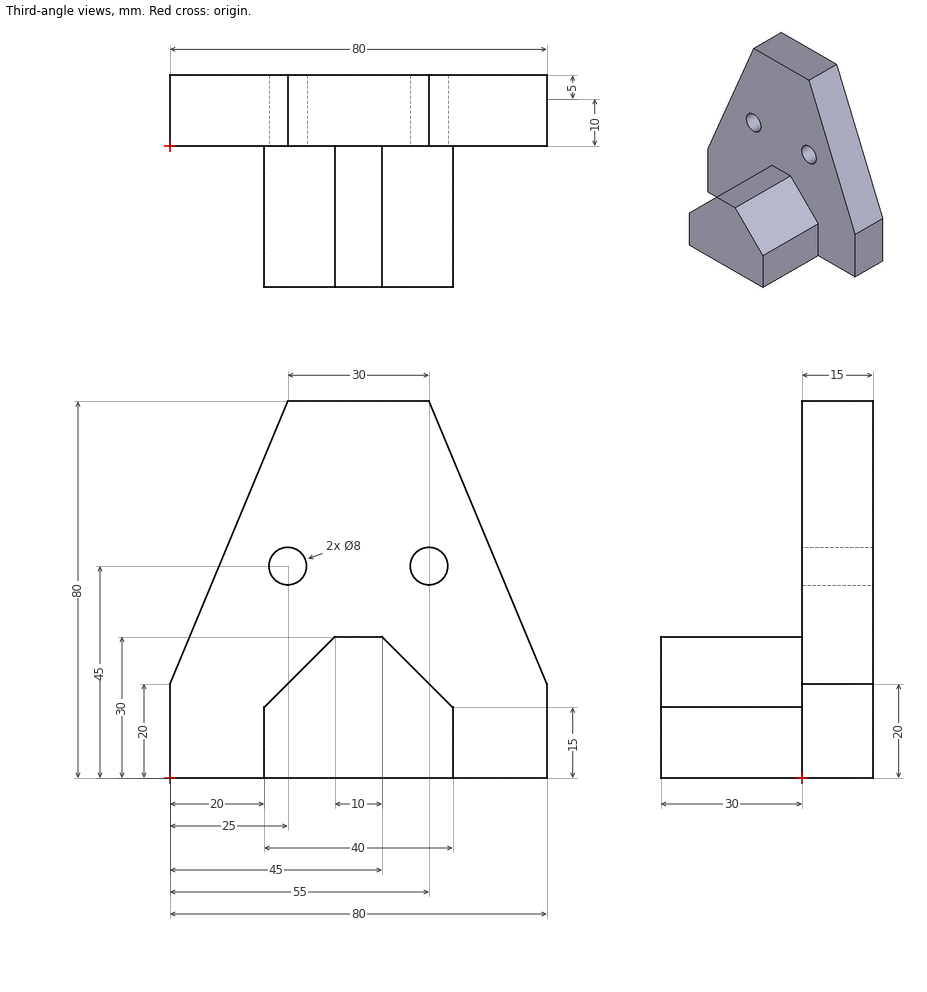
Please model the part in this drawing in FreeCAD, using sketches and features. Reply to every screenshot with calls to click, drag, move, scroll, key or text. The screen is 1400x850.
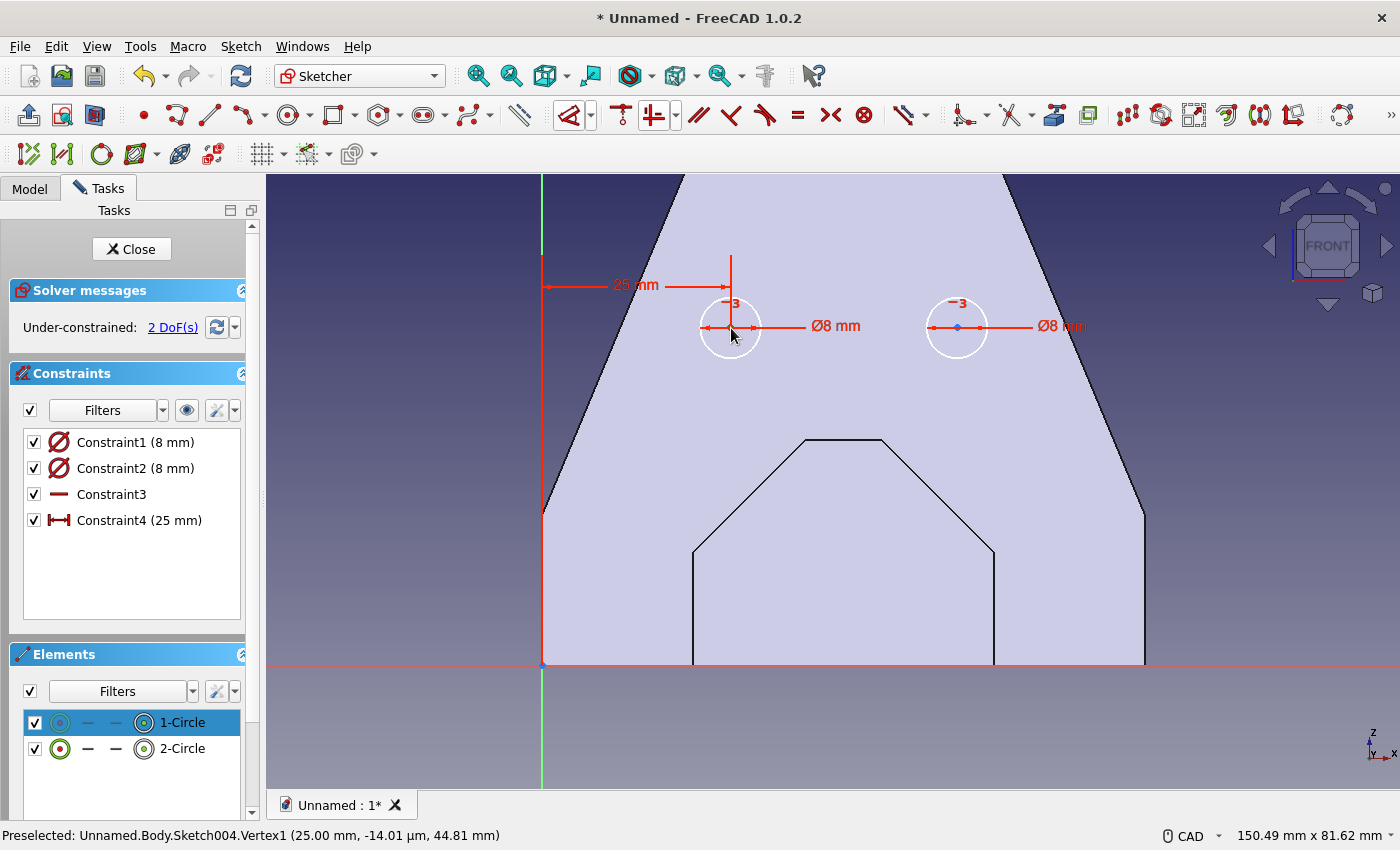
key(i)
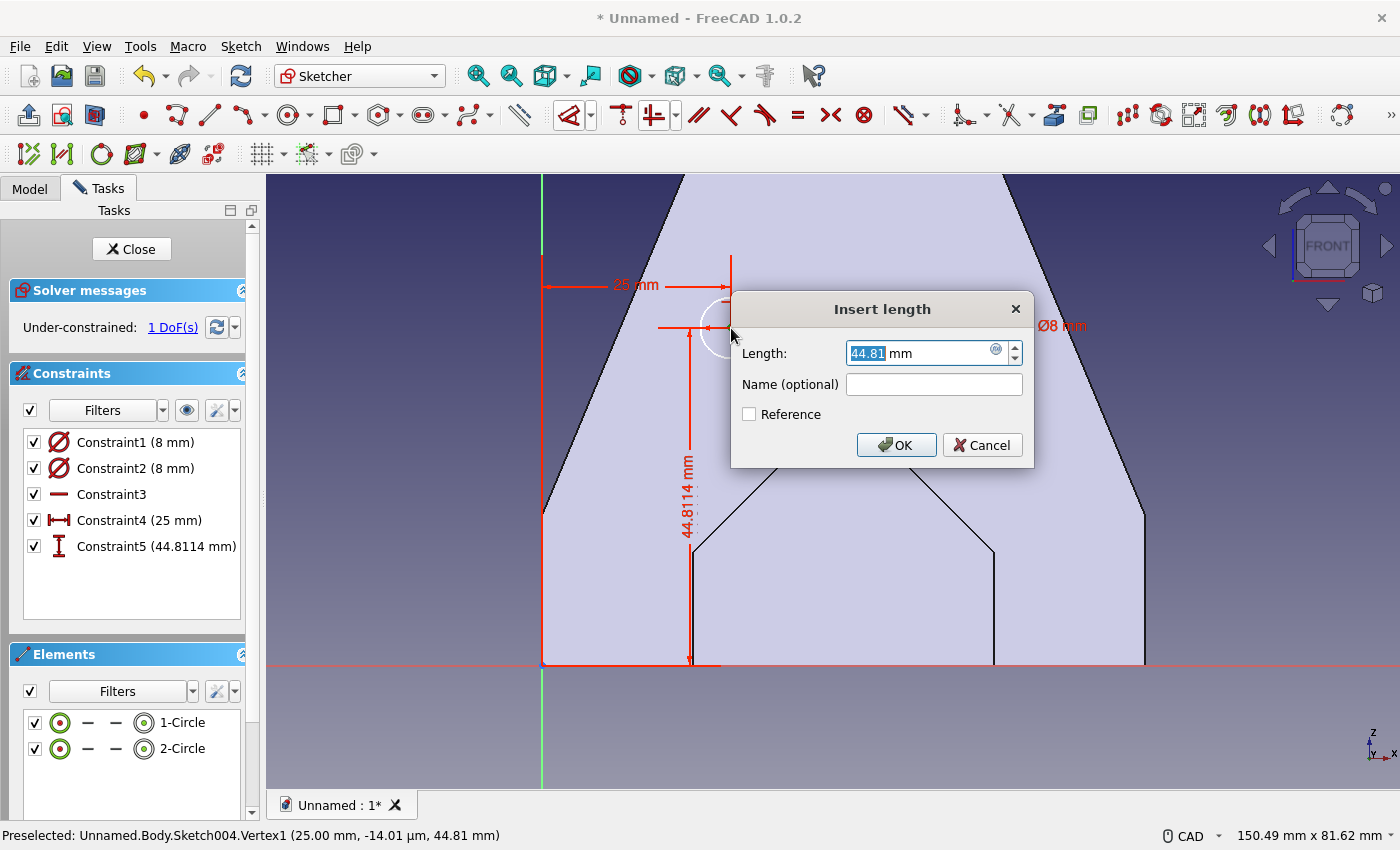
text(45)
key(Return)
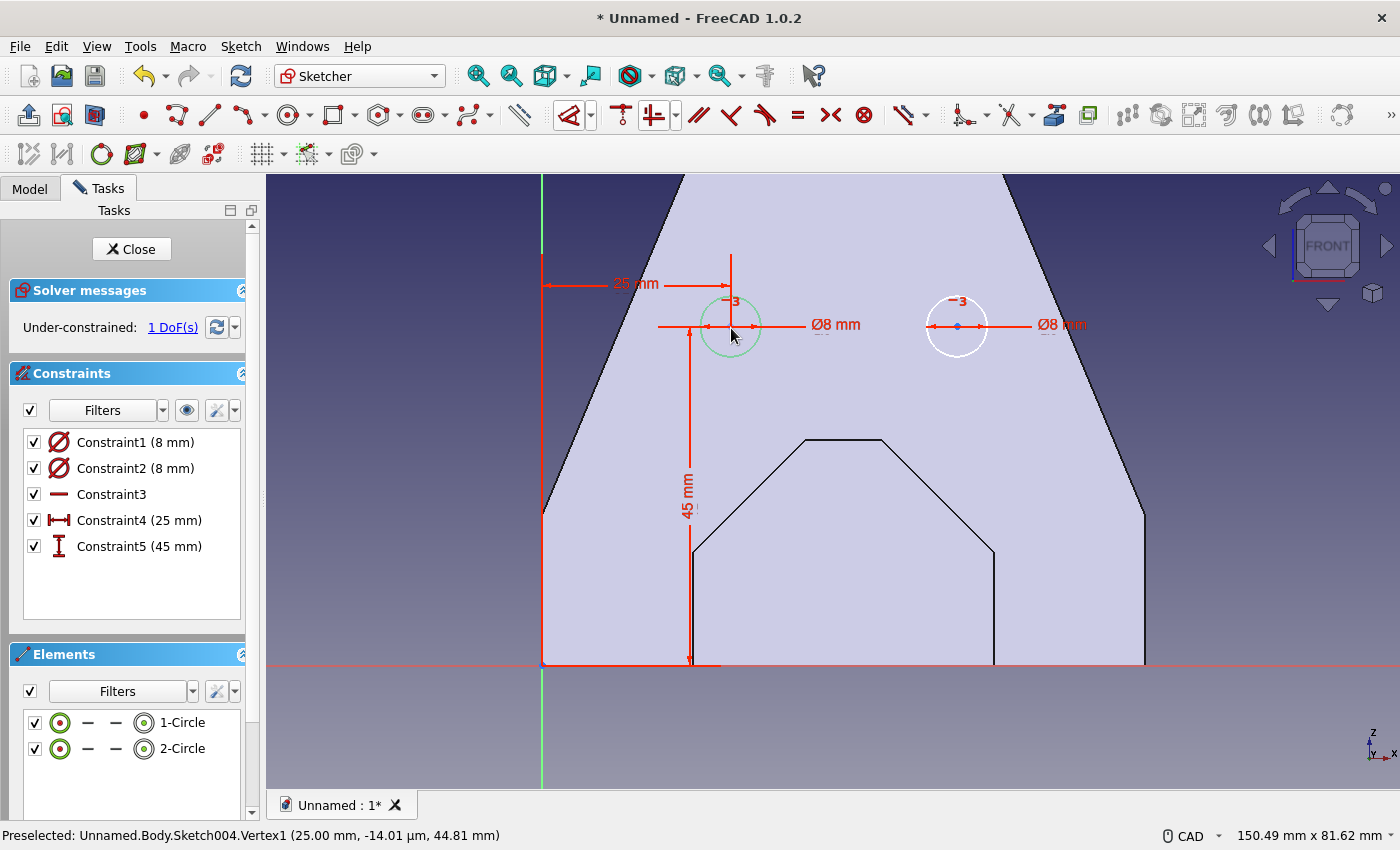
click(957, 327)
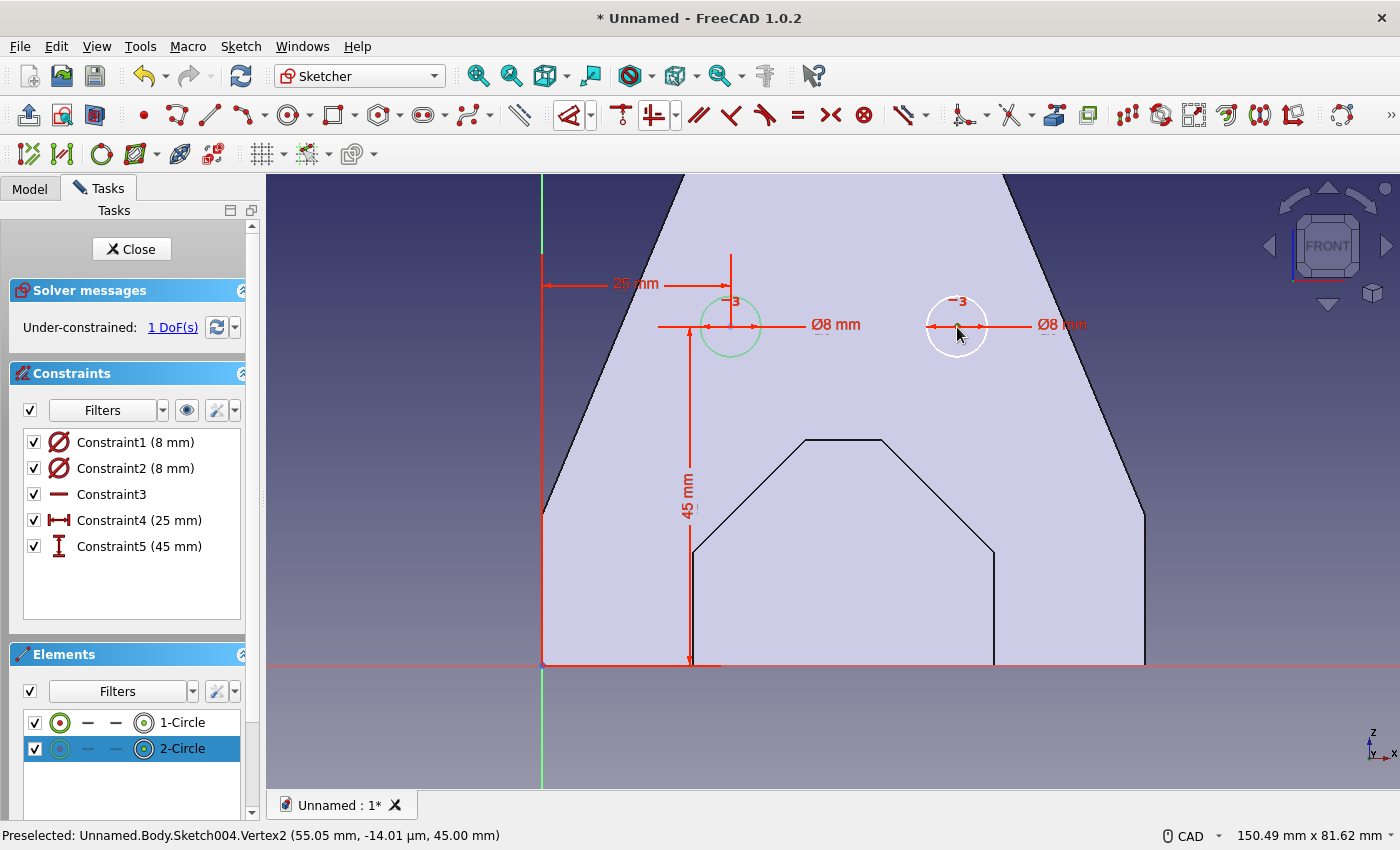
key(l)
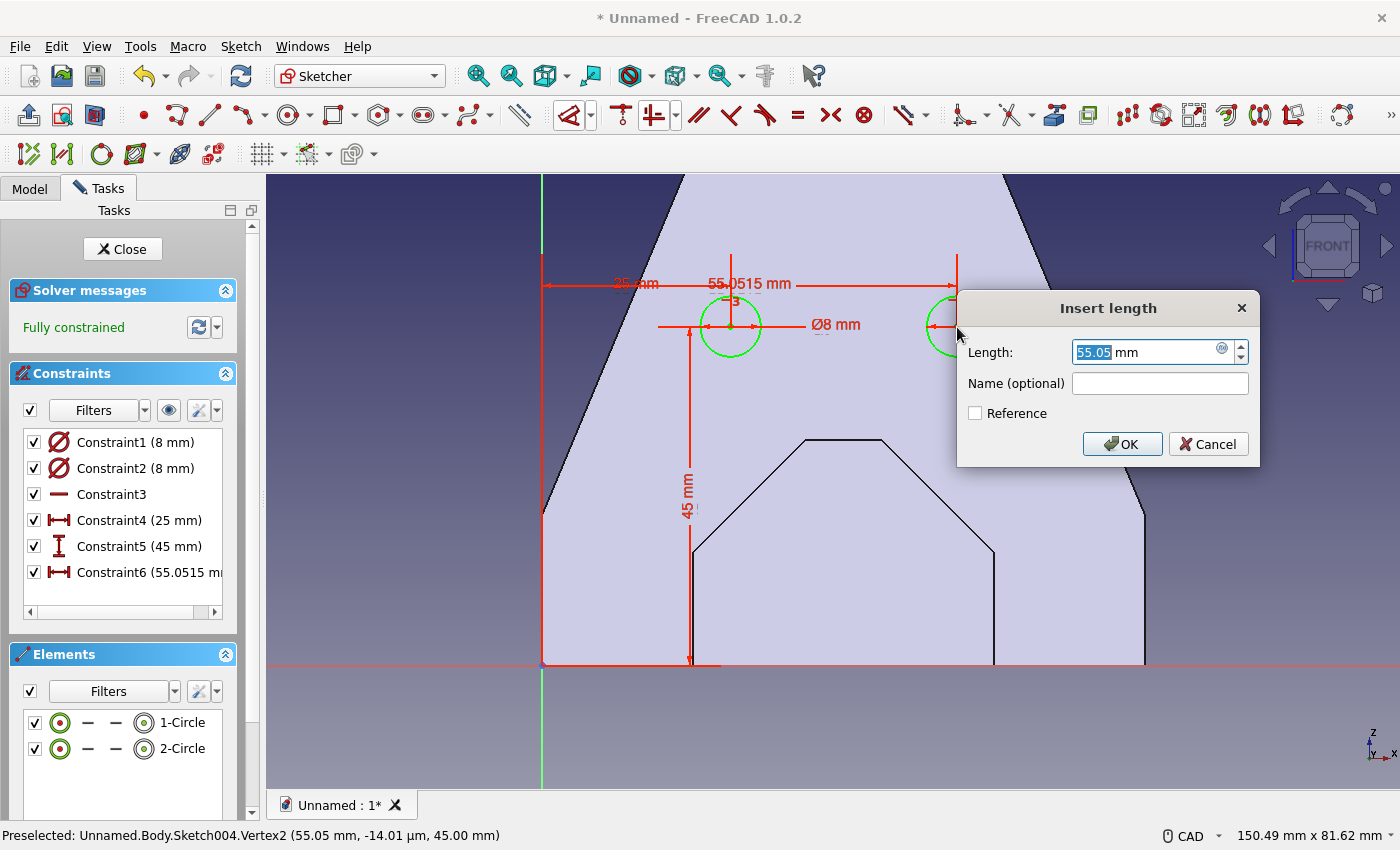
text(55)
key(Return)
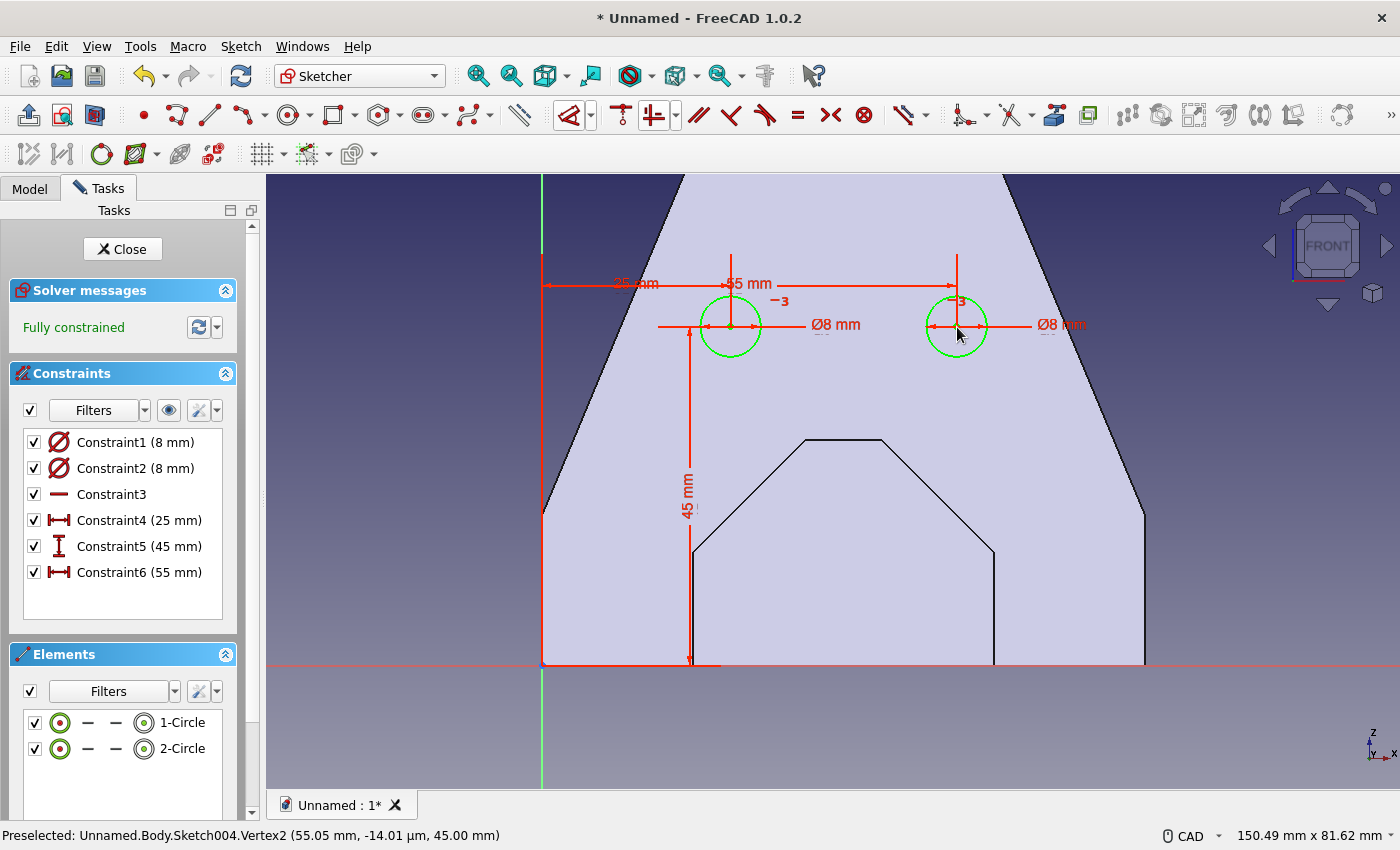
click(123, 249)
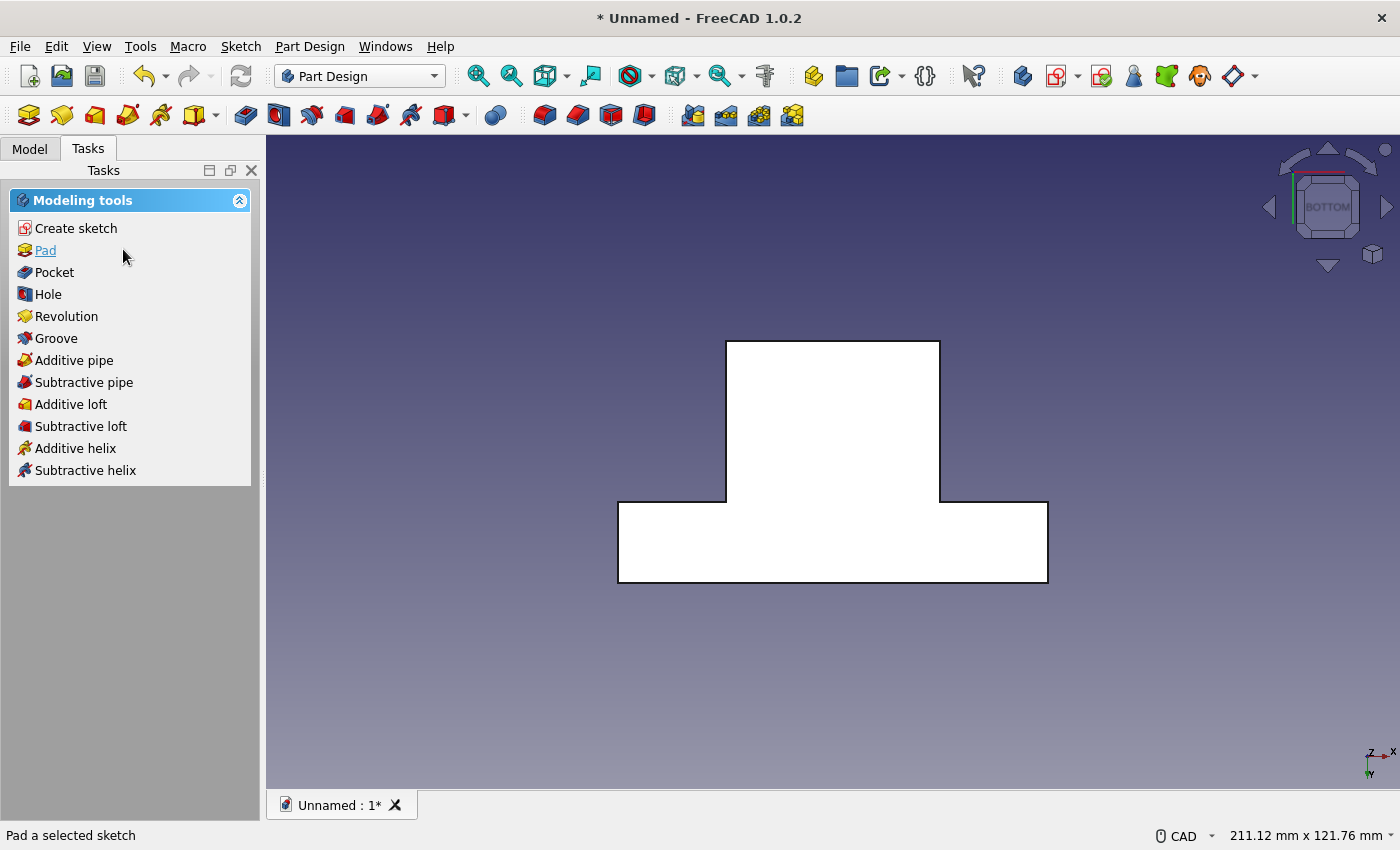
click(246, 116)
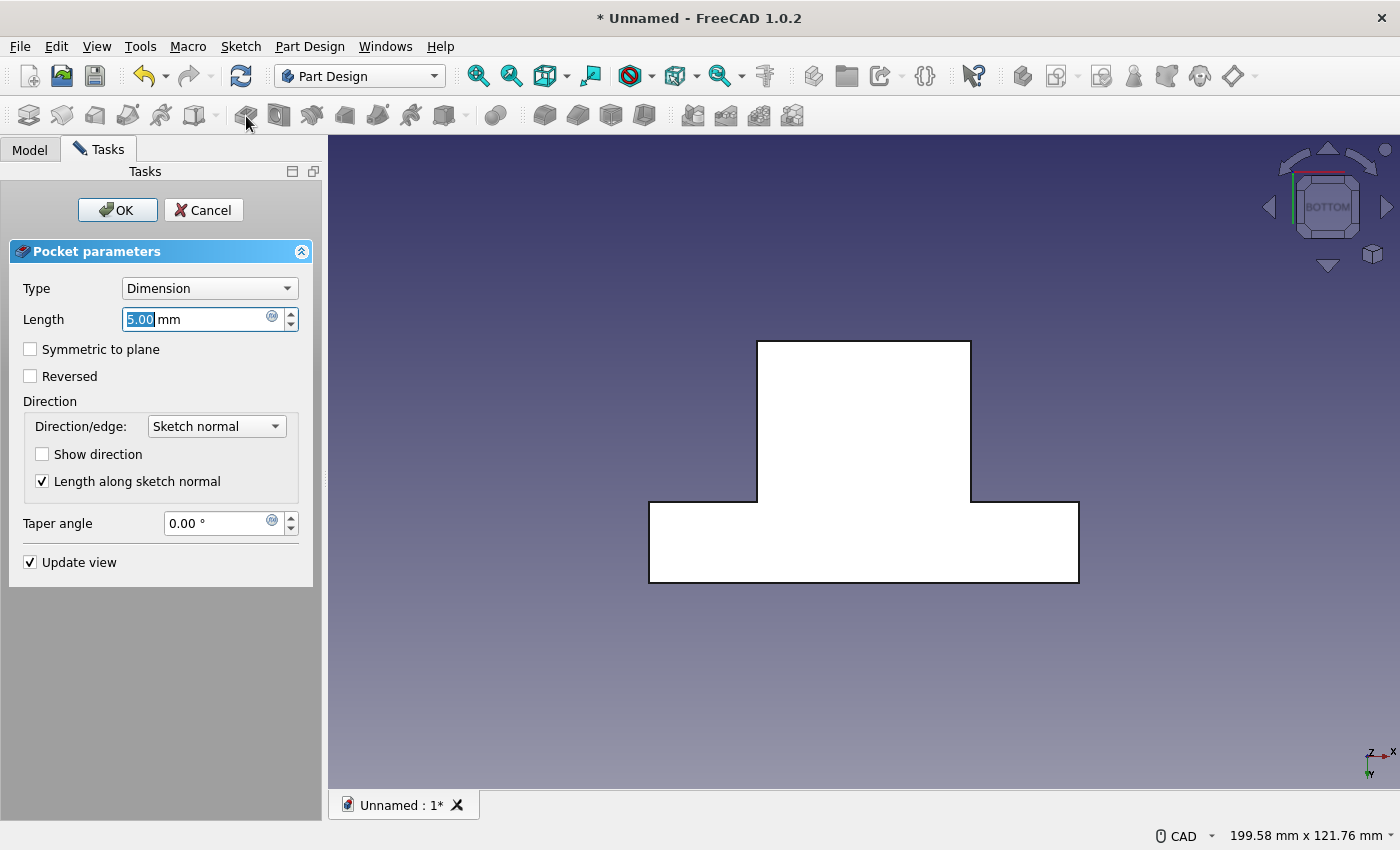
text(15)
key(Tab)